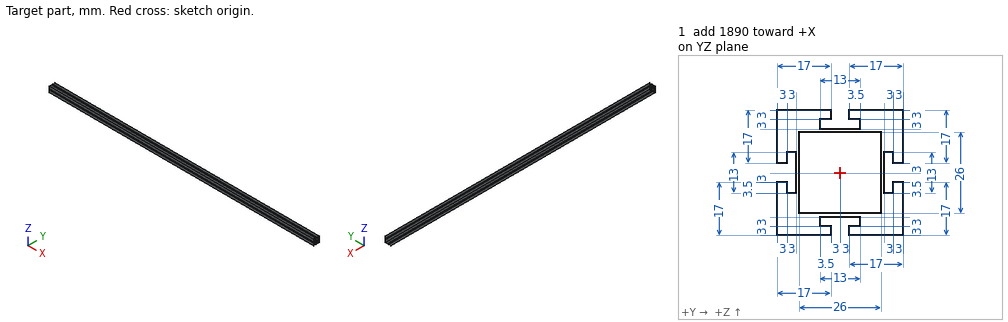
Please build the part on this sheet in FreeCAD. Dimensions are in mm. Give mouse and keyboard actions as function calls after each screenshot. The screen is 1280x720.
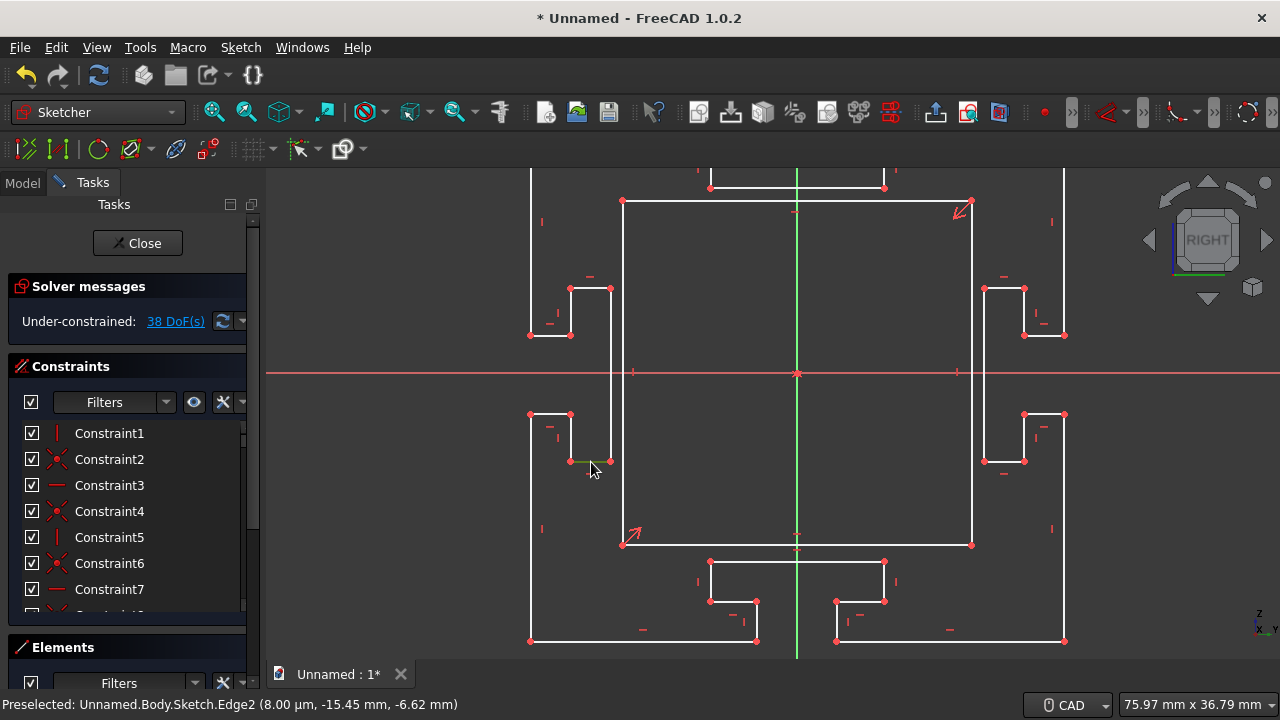
click(1128, 112)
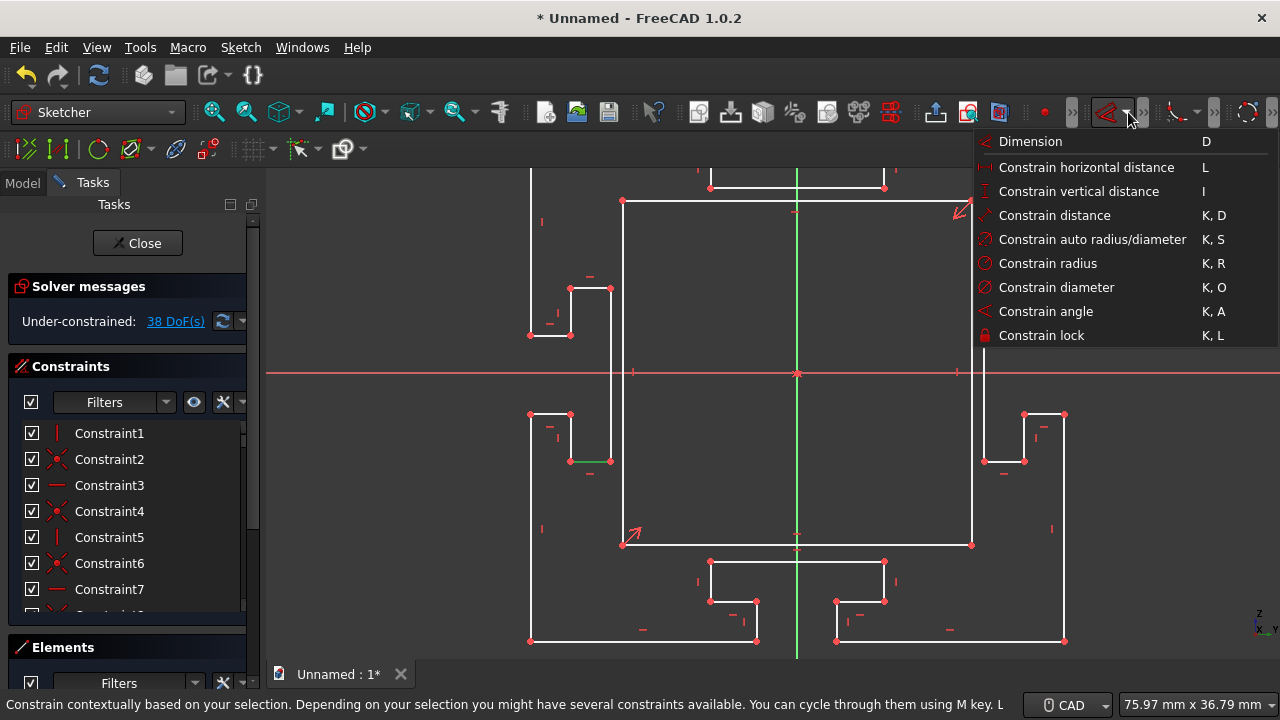
click(1126, 167)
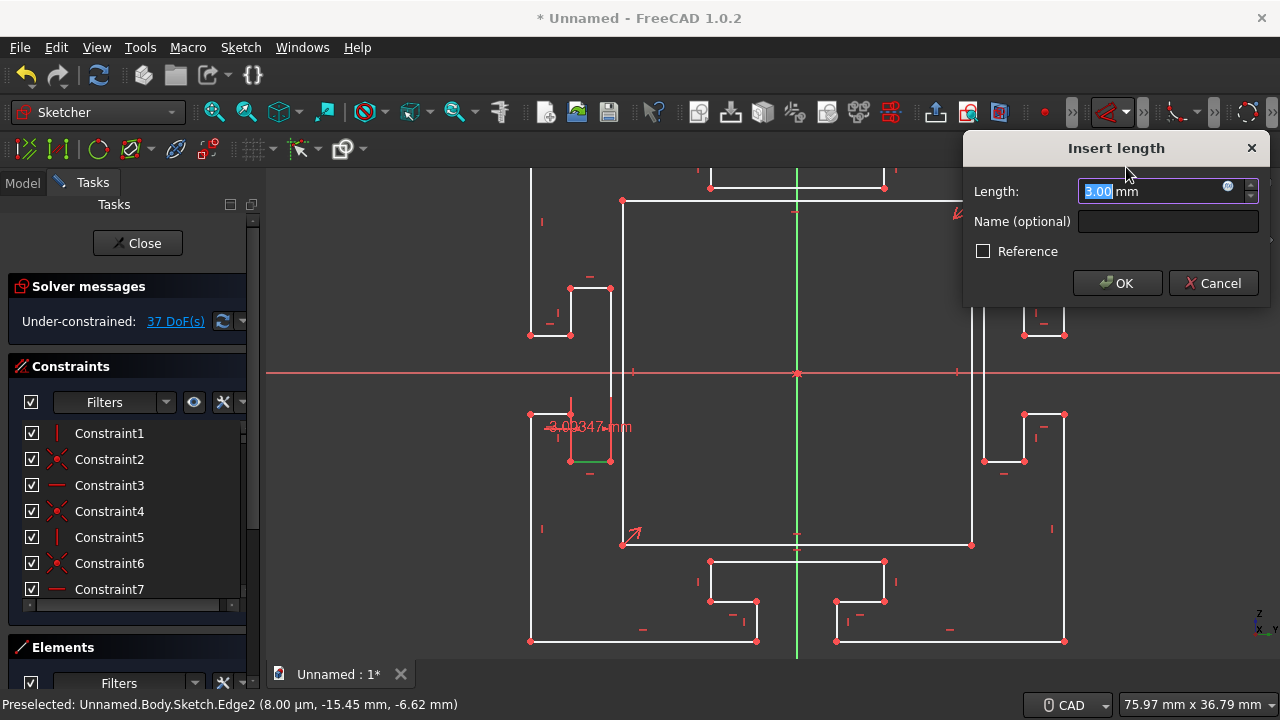
text(3)
key(Return)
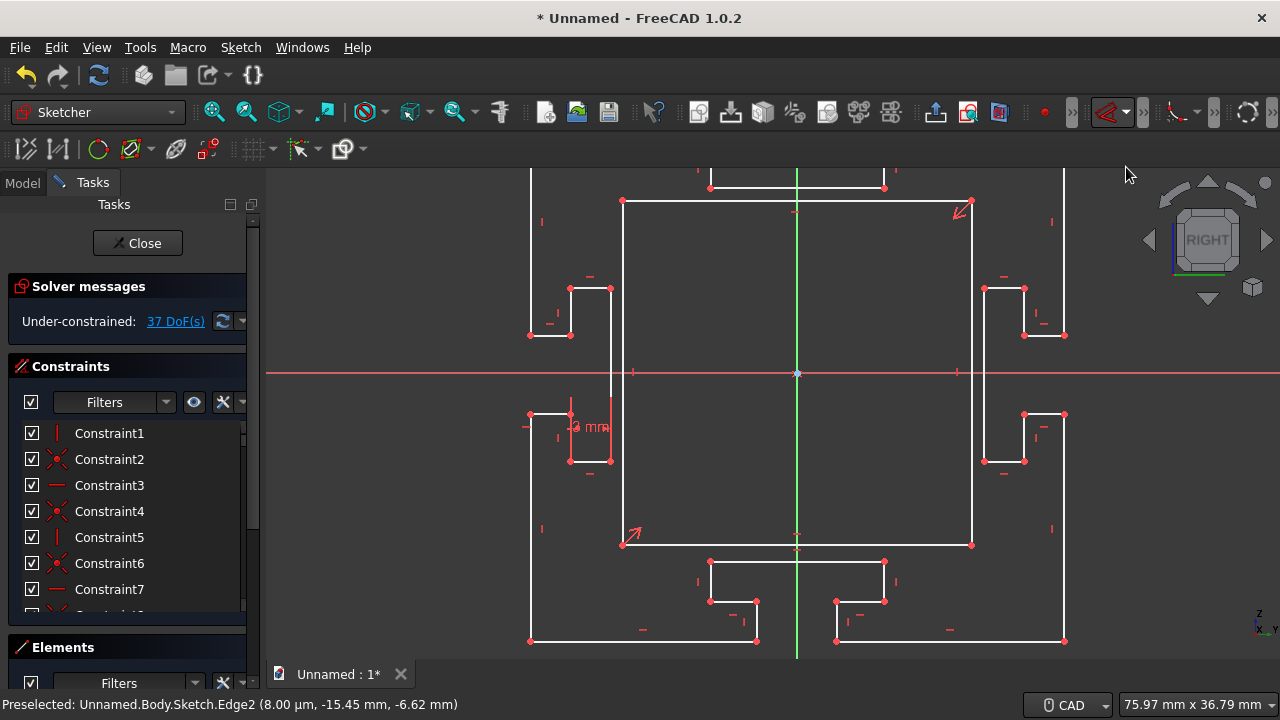
click(559, 414)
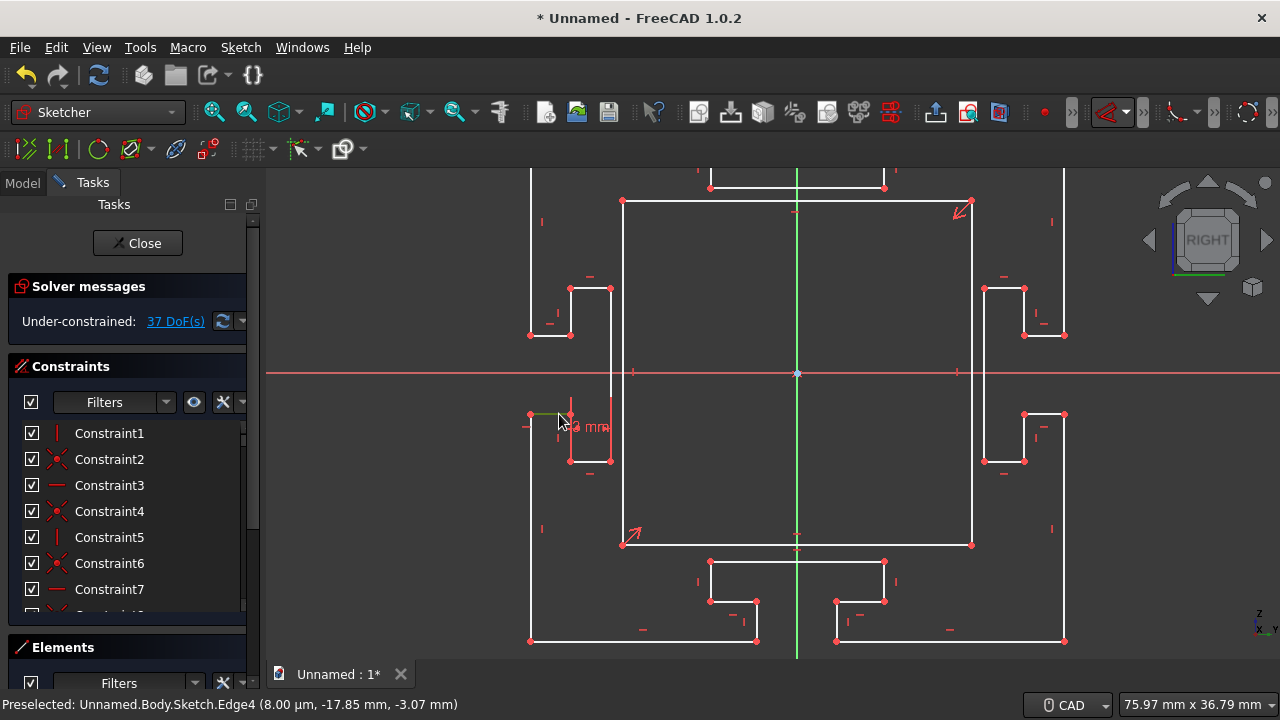
key(l)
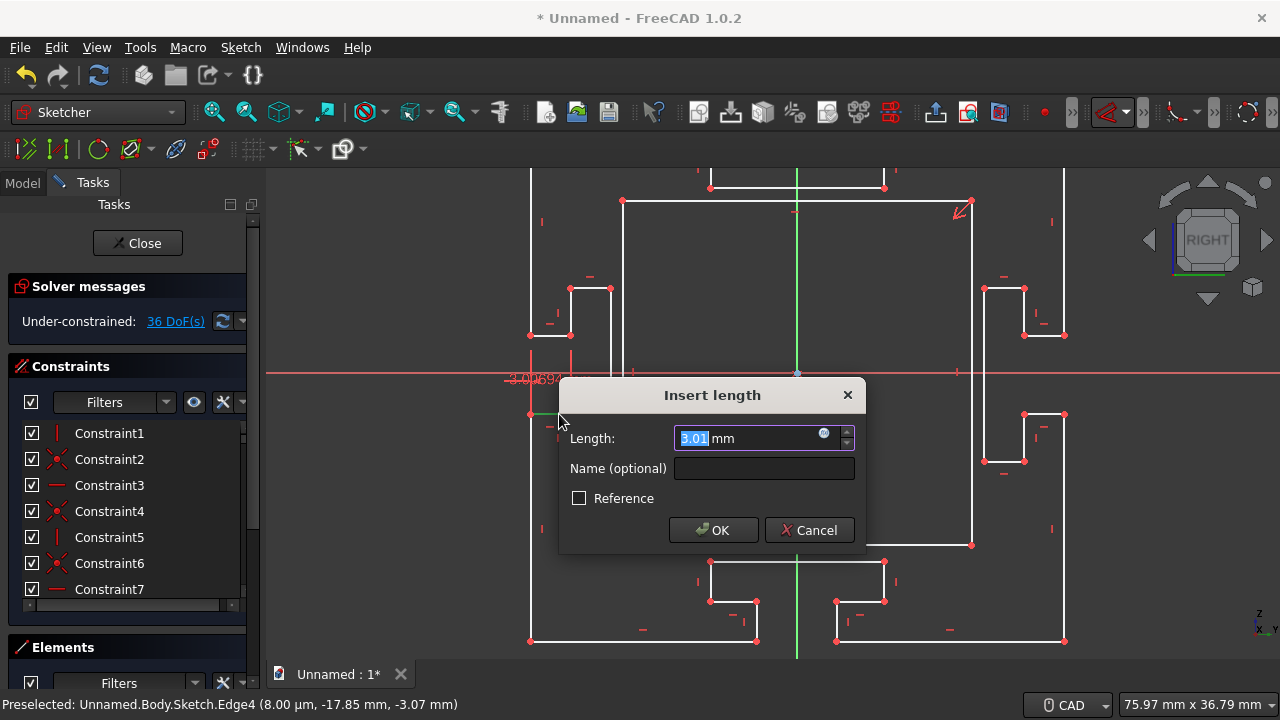
text(3)
key(Return)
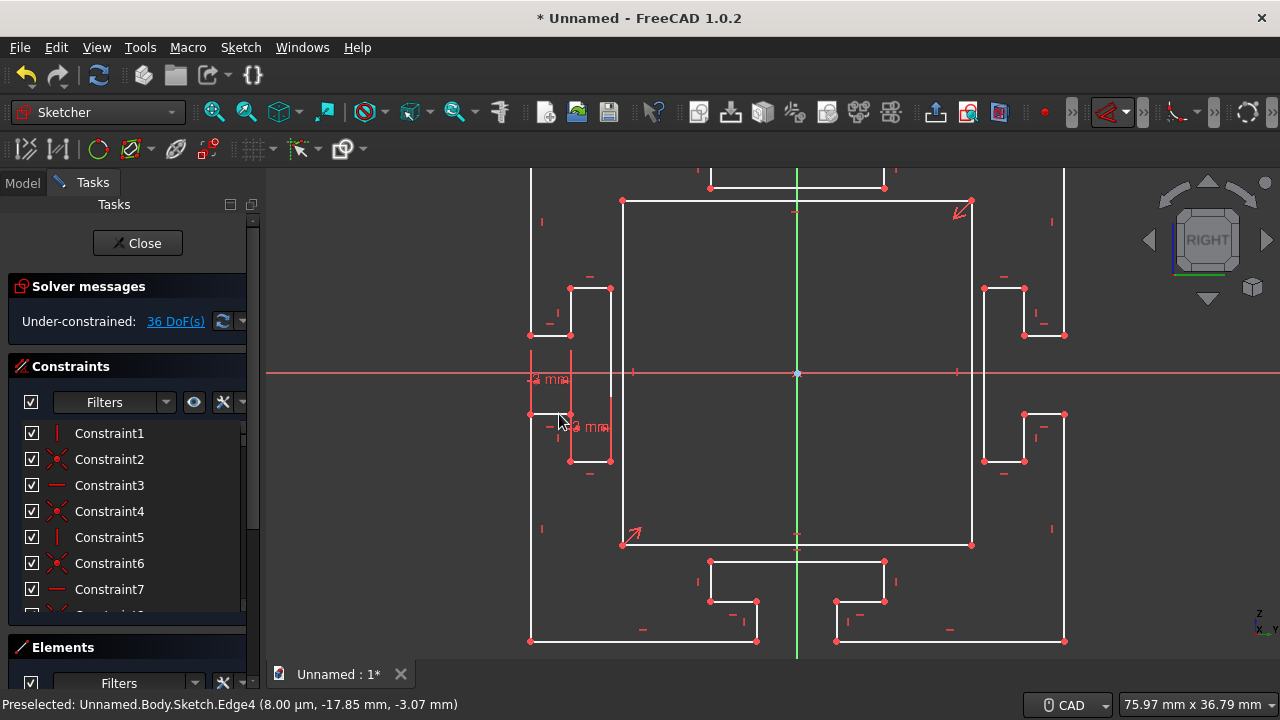
click(757, 630)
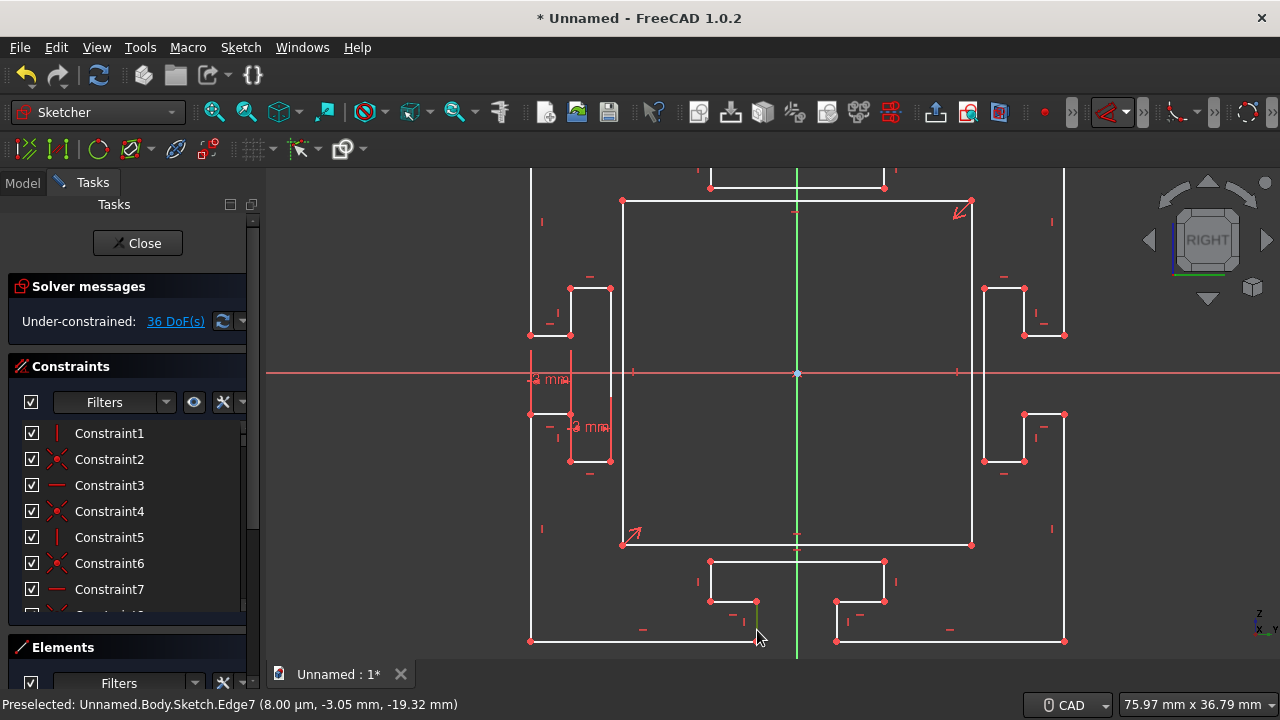
key(i)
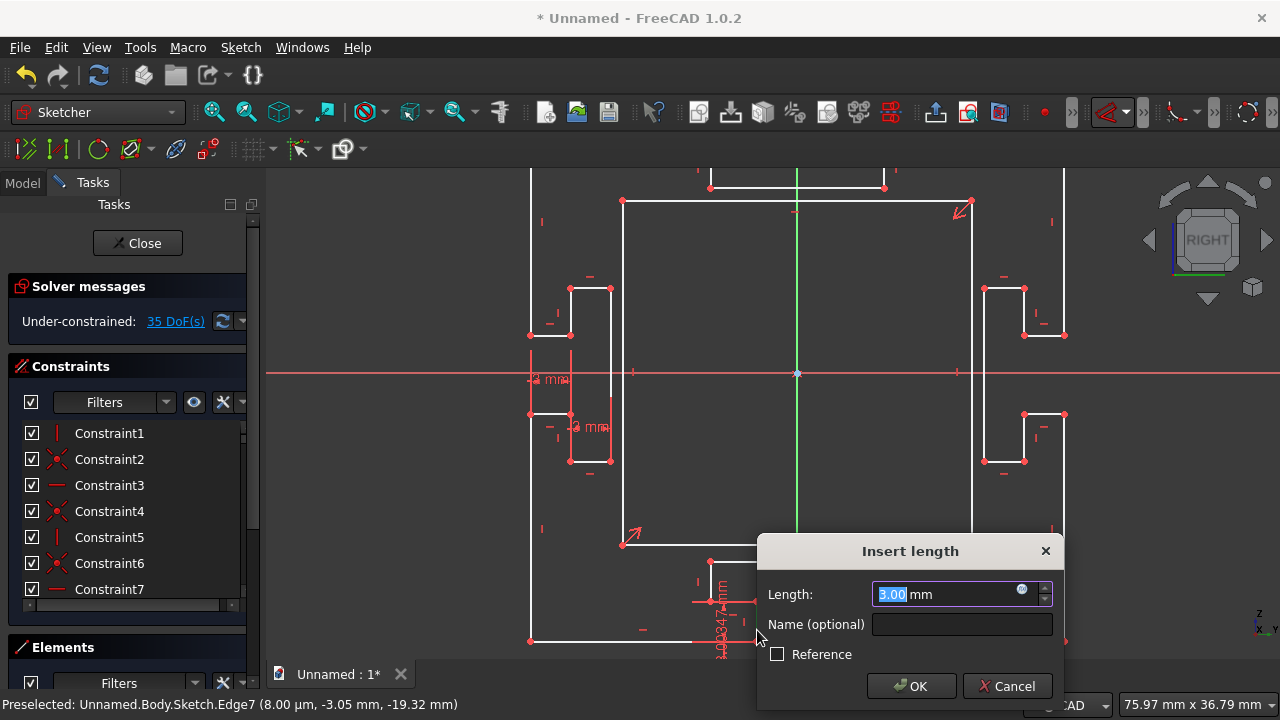
text(3)
key(Return)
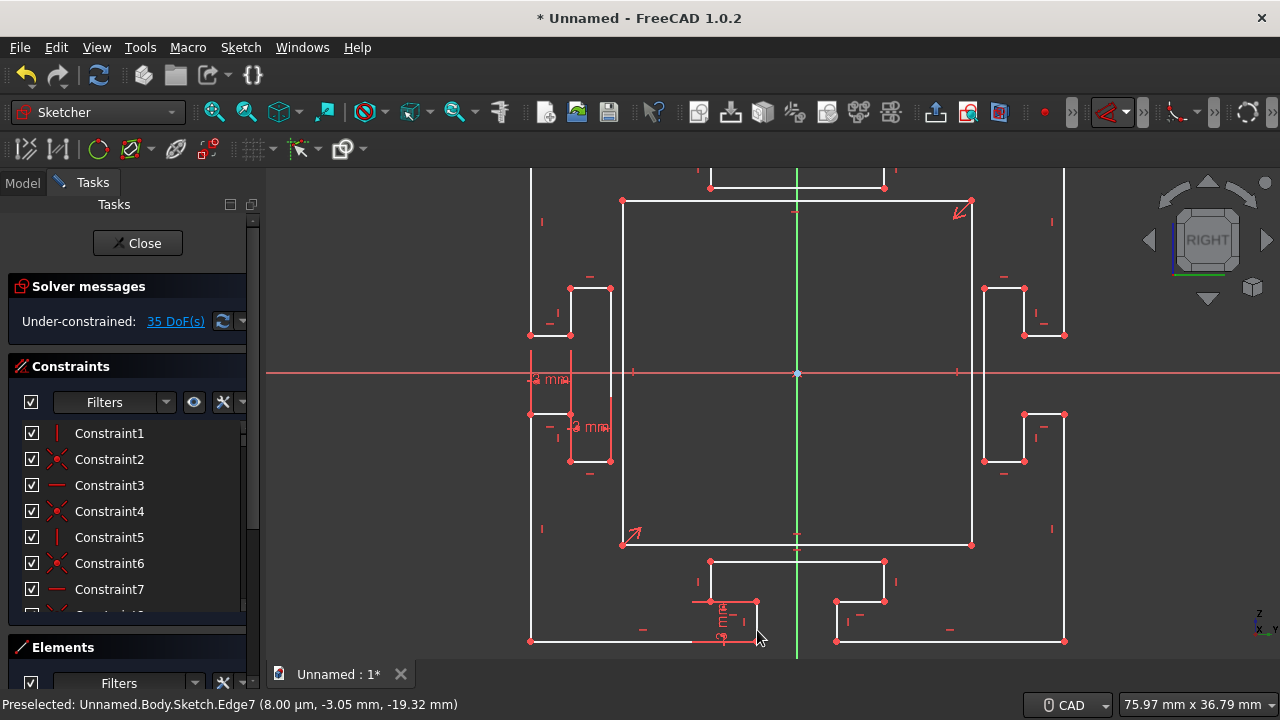
click(711, 590)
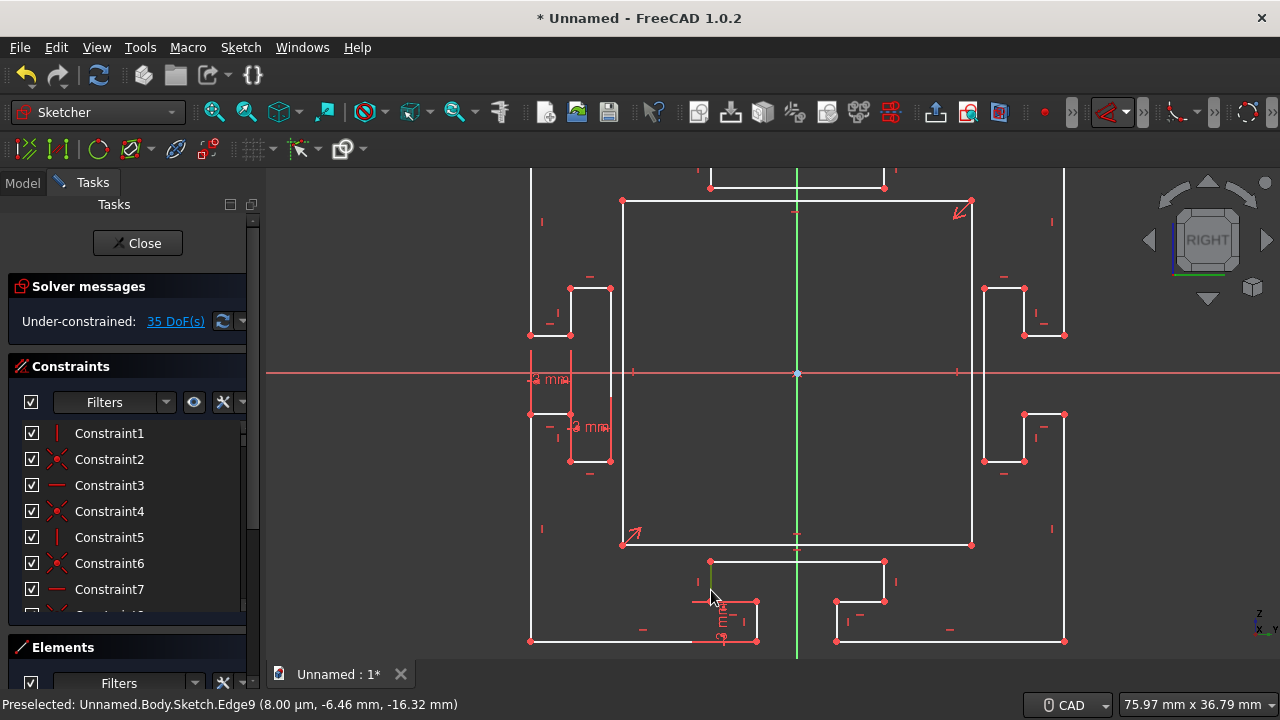
click(1128, 112)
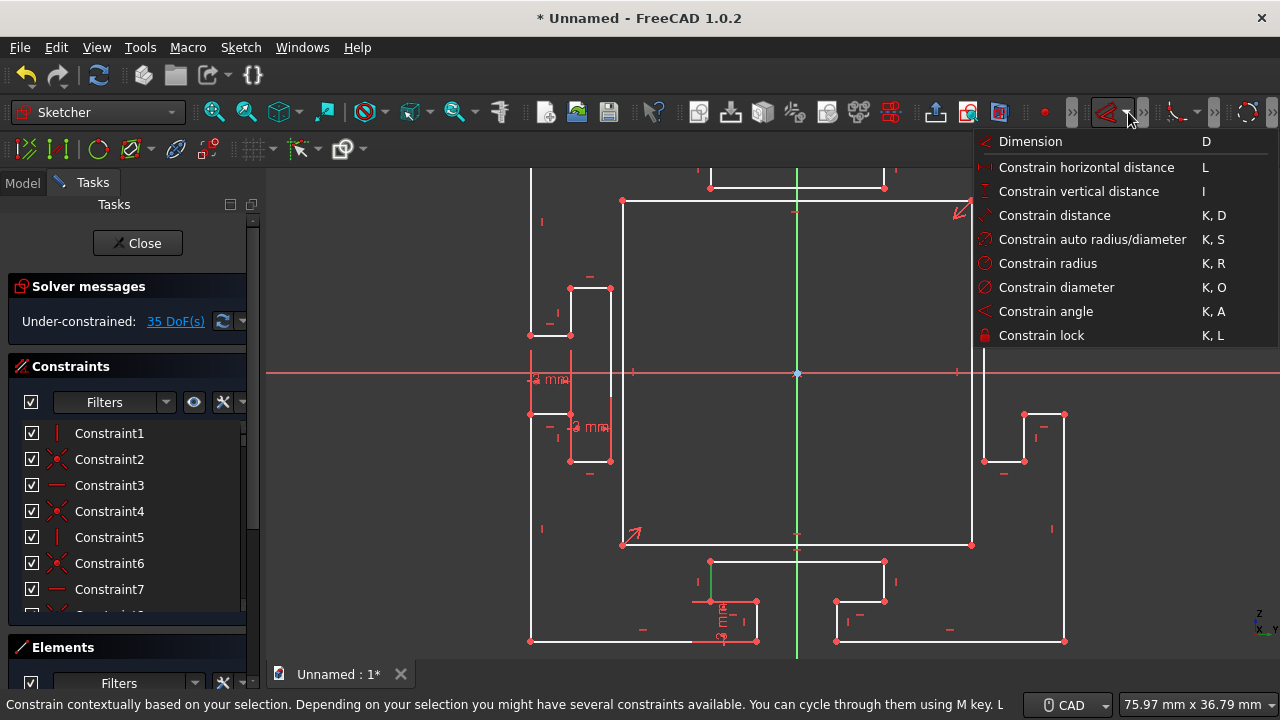
click(1126, 191)